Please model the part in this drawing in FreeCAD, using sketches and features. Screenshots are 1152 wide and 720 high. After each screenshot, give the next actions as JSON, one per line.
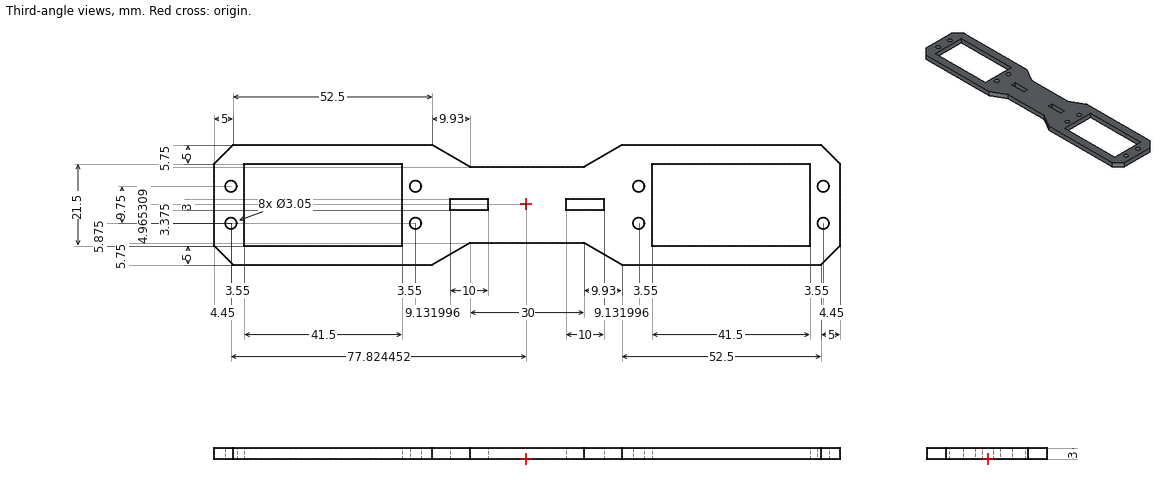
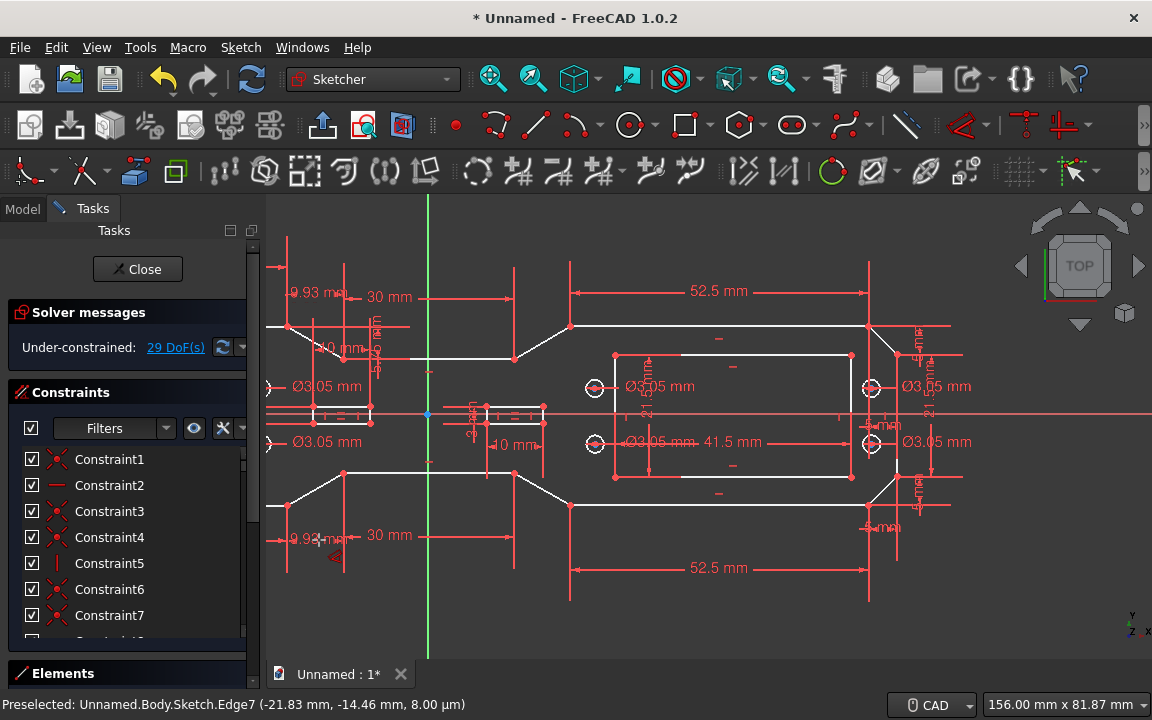
{"action": "left_click", "coordinate": [304, 496]}
{"action": "left_click", "coordinate": [378, 489]}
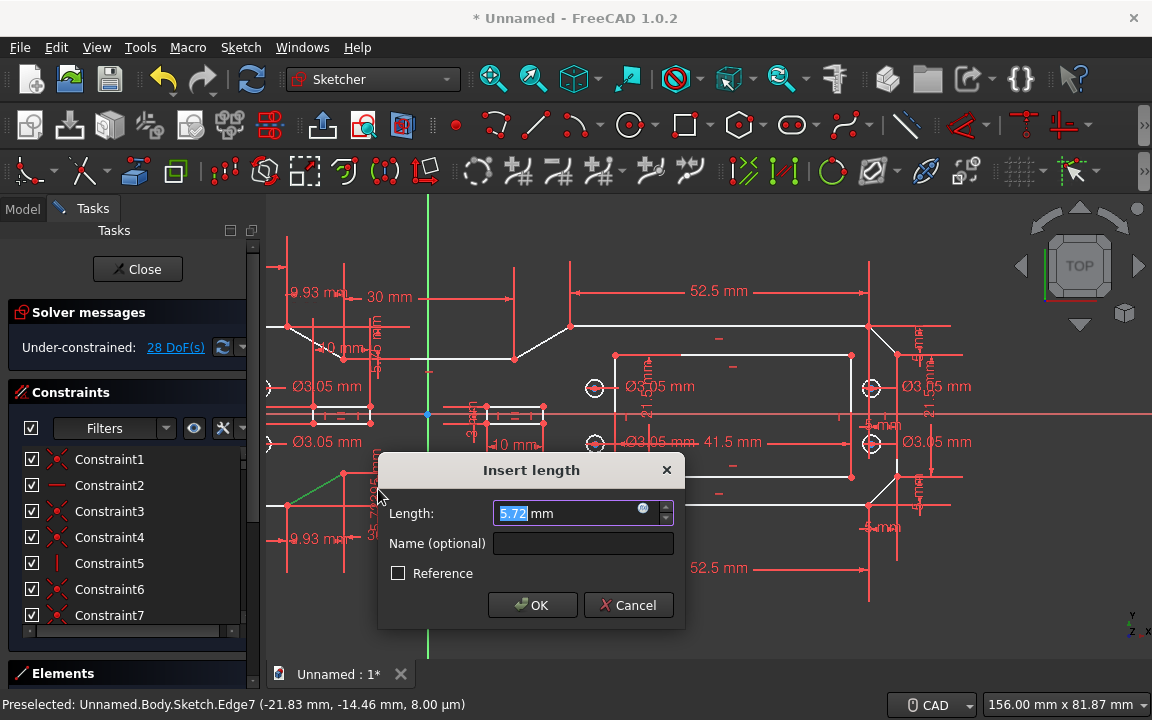
{"action": "type", "text": "5.75"}
{"action": "key", "text": "Return"}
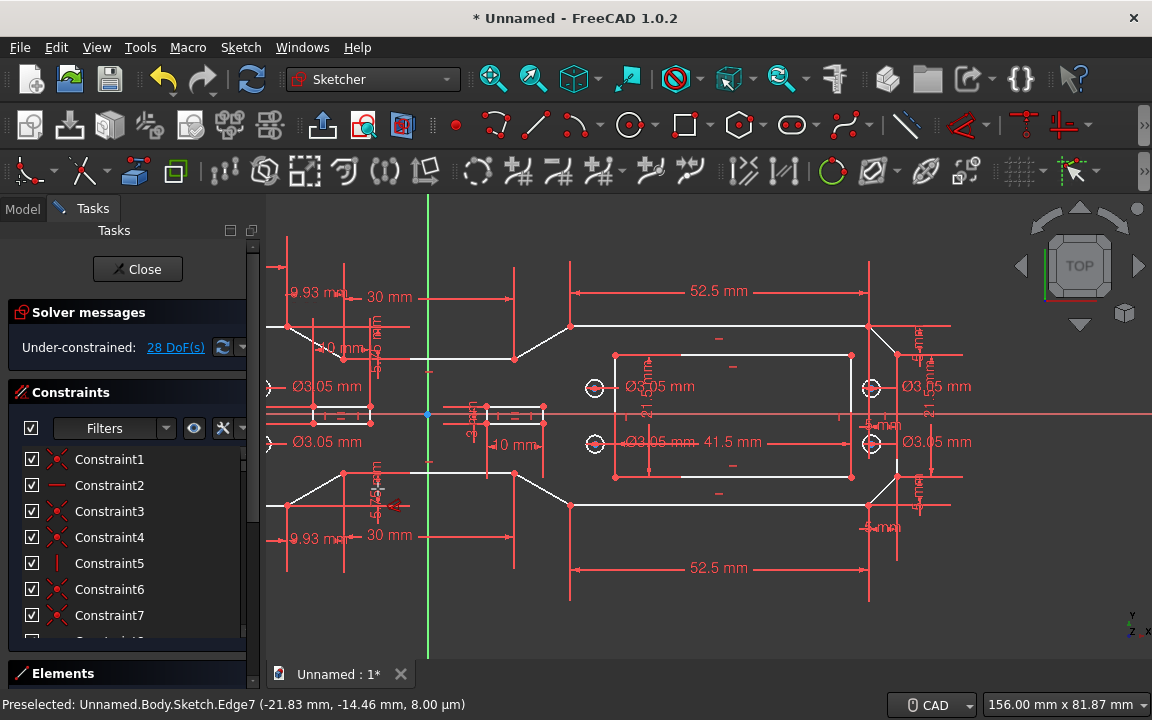
{"action": "left_click", "coordinate": [531, 483]}
{"action": "left_click", "coordinate": [542, 539]}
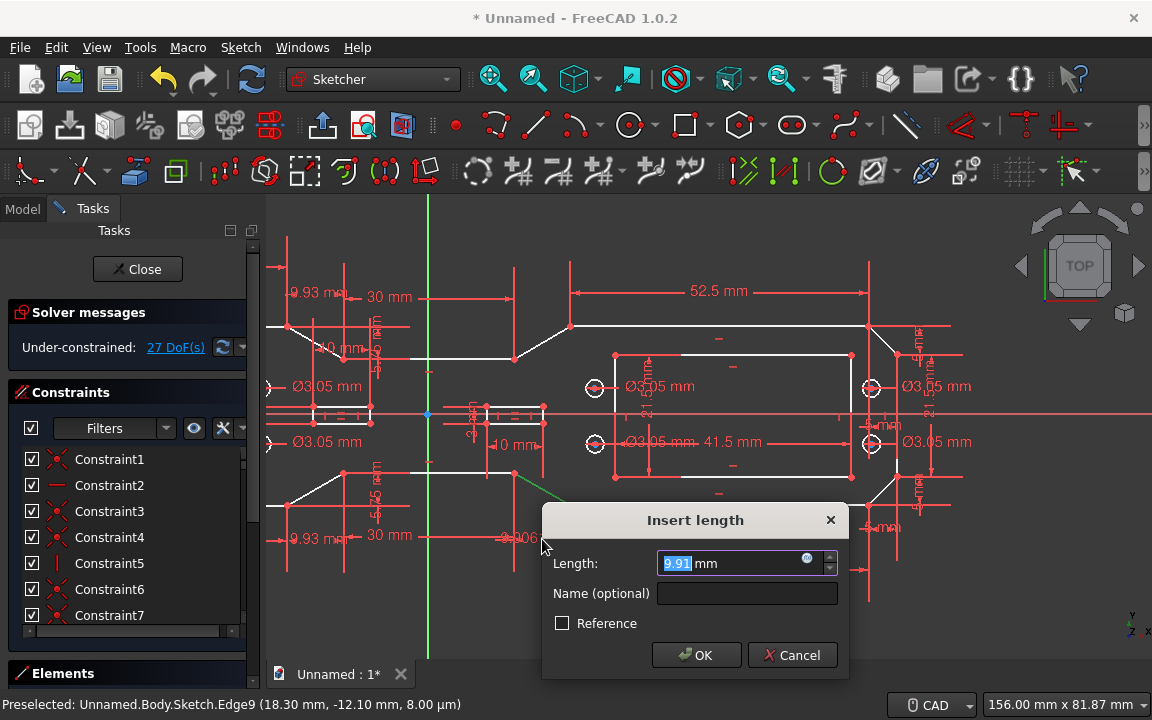
{"action": "type", "text": "9.93"}
{"action": "key", "text": "Return"}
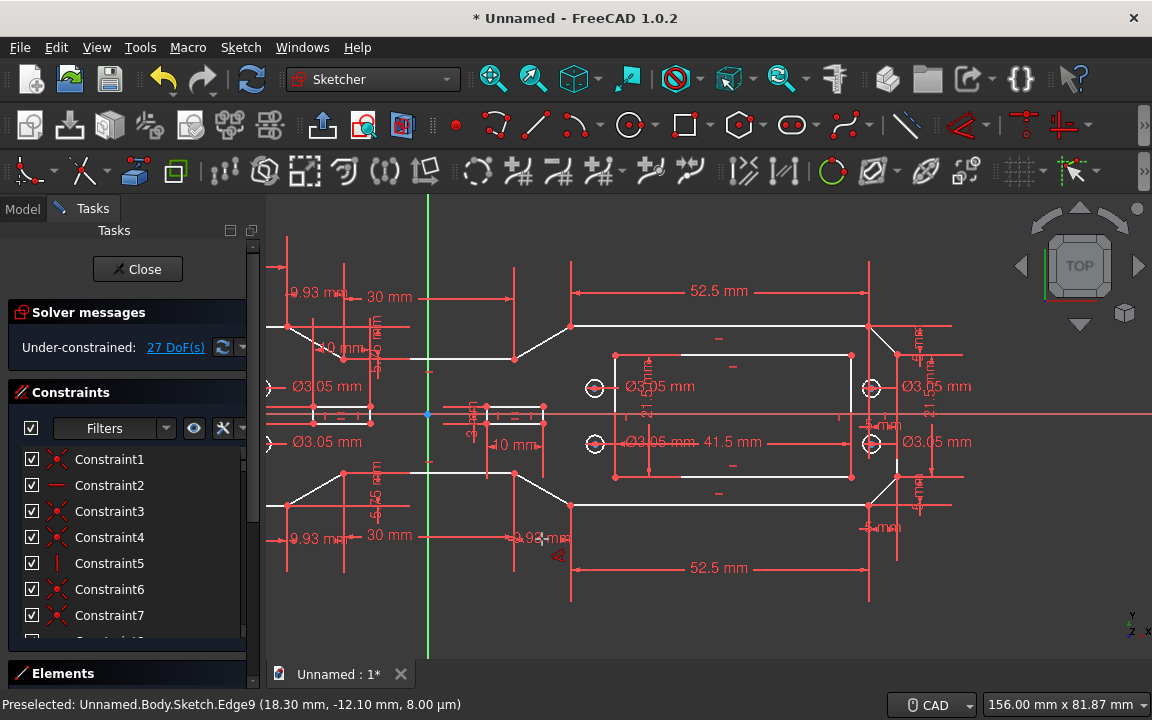
{"action": "left_click", "coordinate": [531, 483]}
{"action": "left_click", "coordinate": [605, 489]}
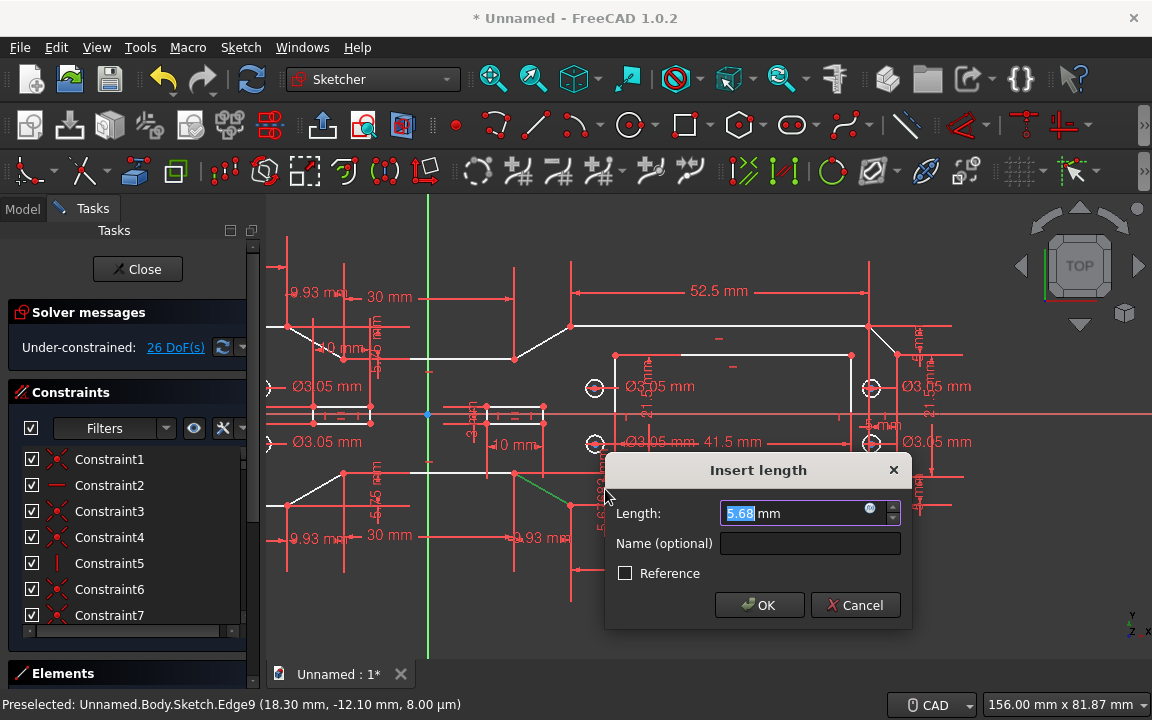
{"action": "type", "text": "5.75"}
{"action": "key", "text": "Return"}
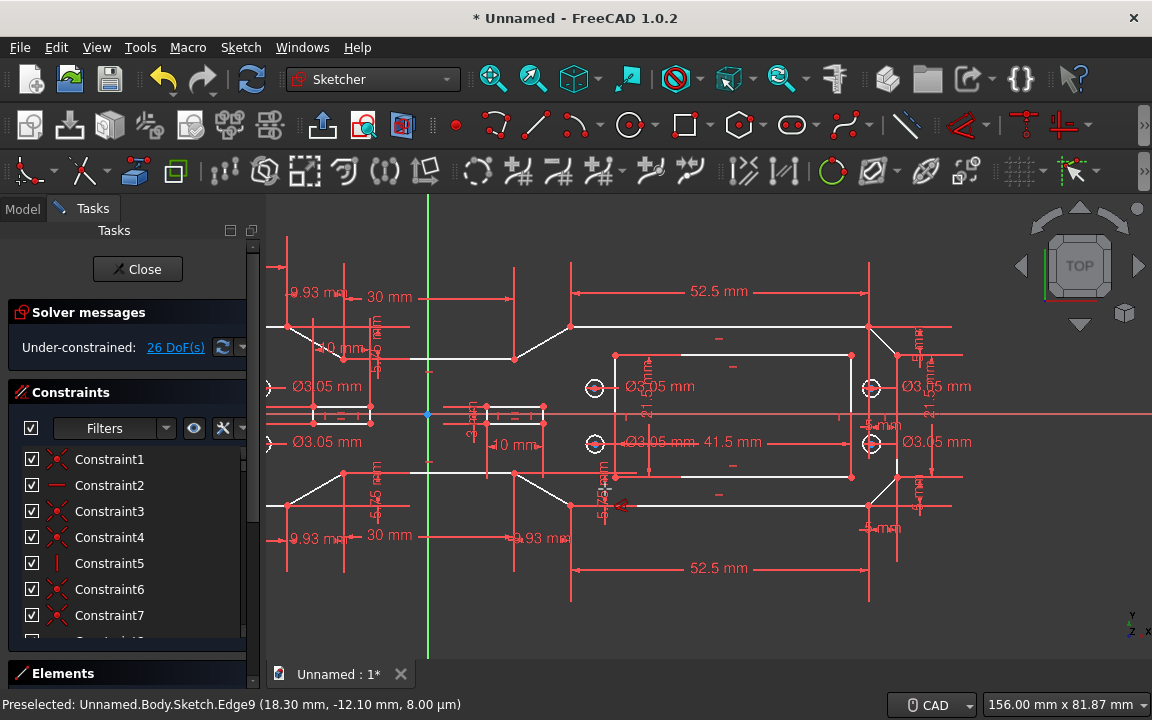
{"action": "scroll", "coordinate": [898, 441], "scroll_direction": "down", "scroll_amount": 3}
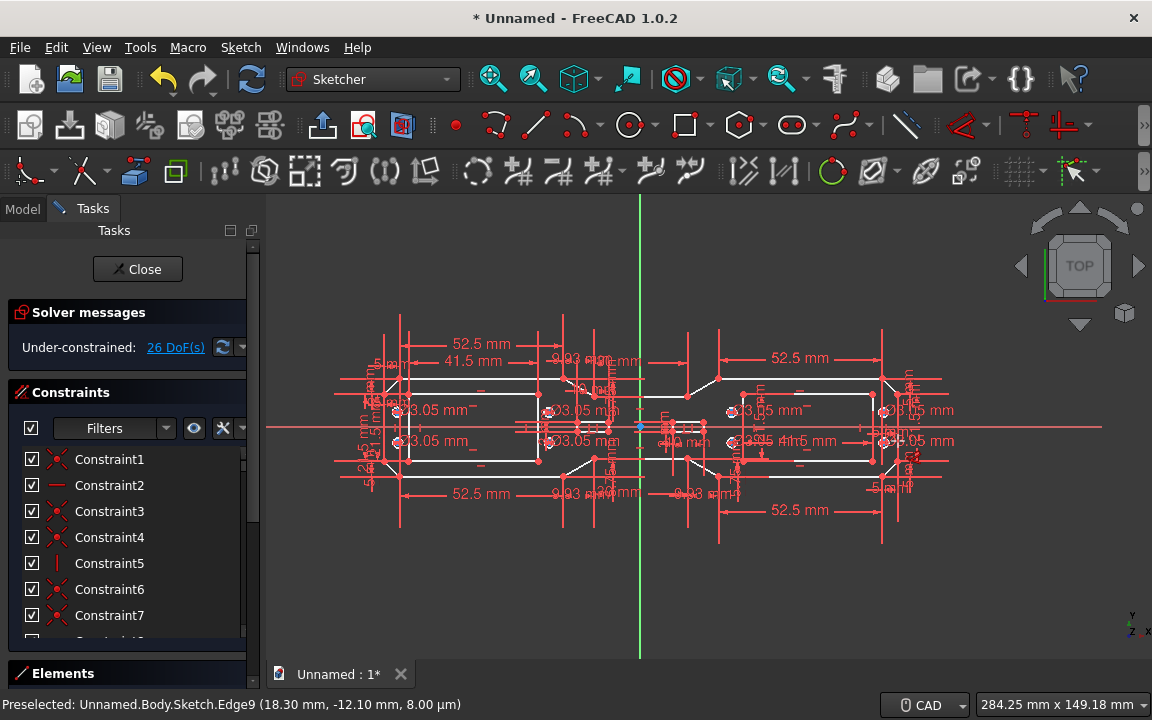
{"action": "scroll", "coordinate": [409, 461], "scroll_direction": "up", "scroll_amount": 7}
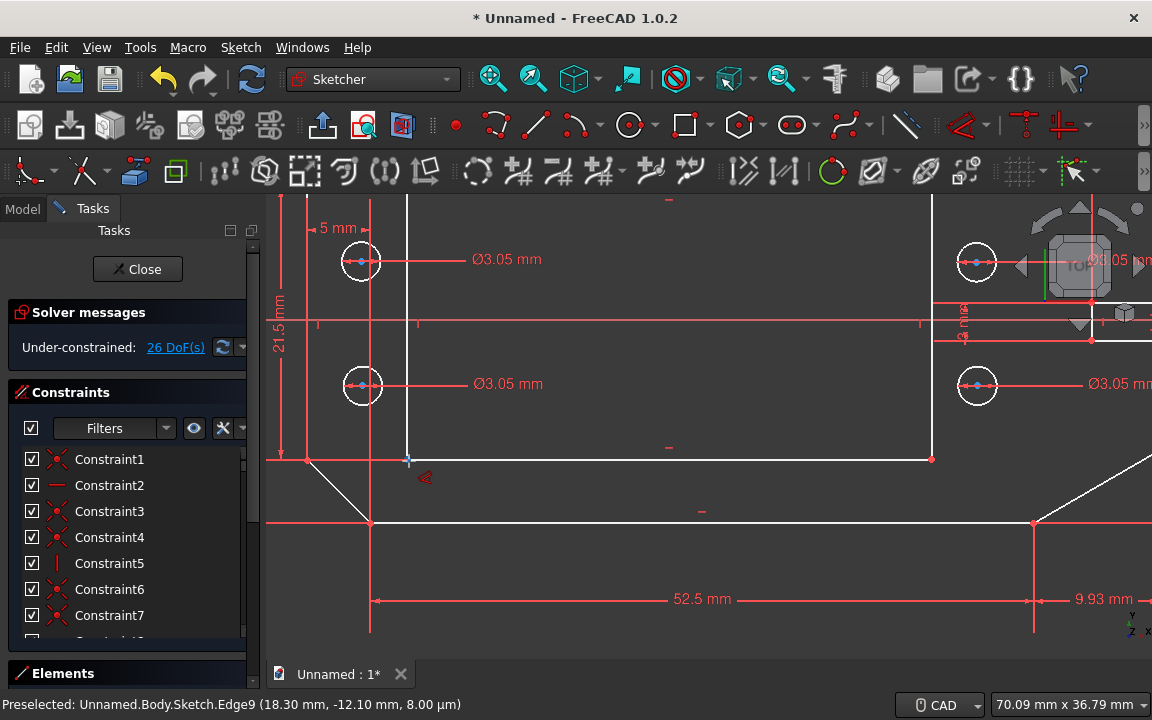
{"action": "left_click", "coordinate": [407, 460]}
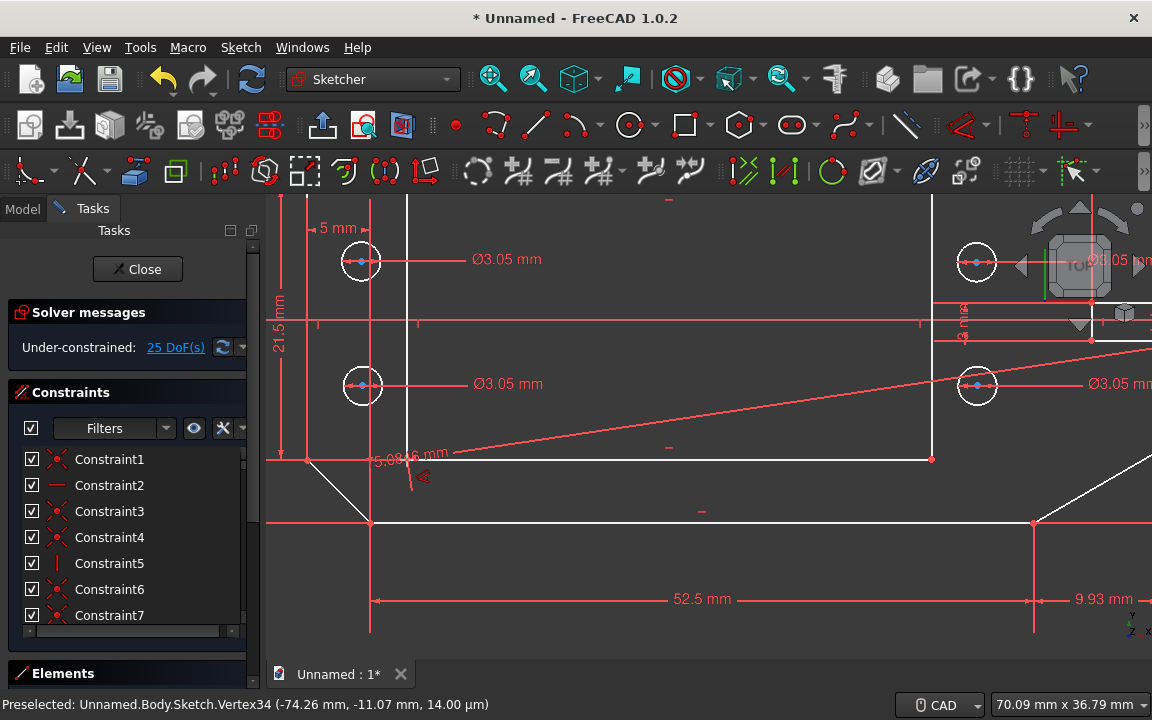
{"action": "left_click", "coordinate": [363, 386]}
{"action": "left_click", "coordinate": [385, 494]}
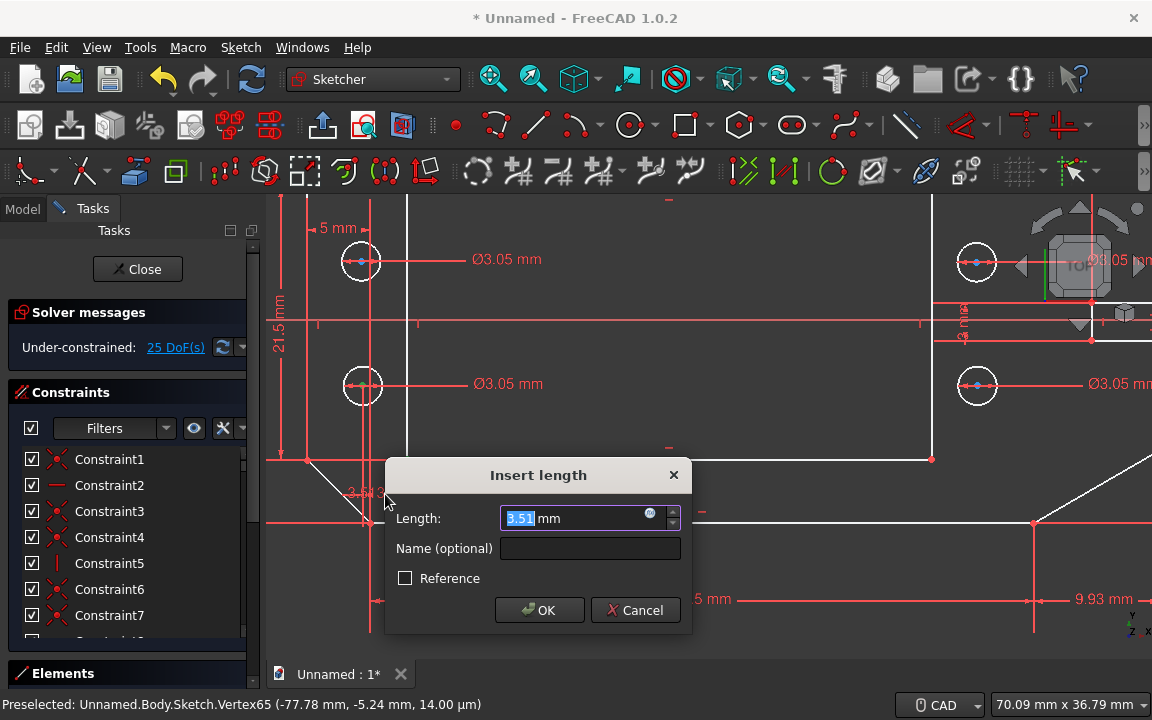
{"action": "type", "text": "3.55"}
{"action": "key", "text": "Return"}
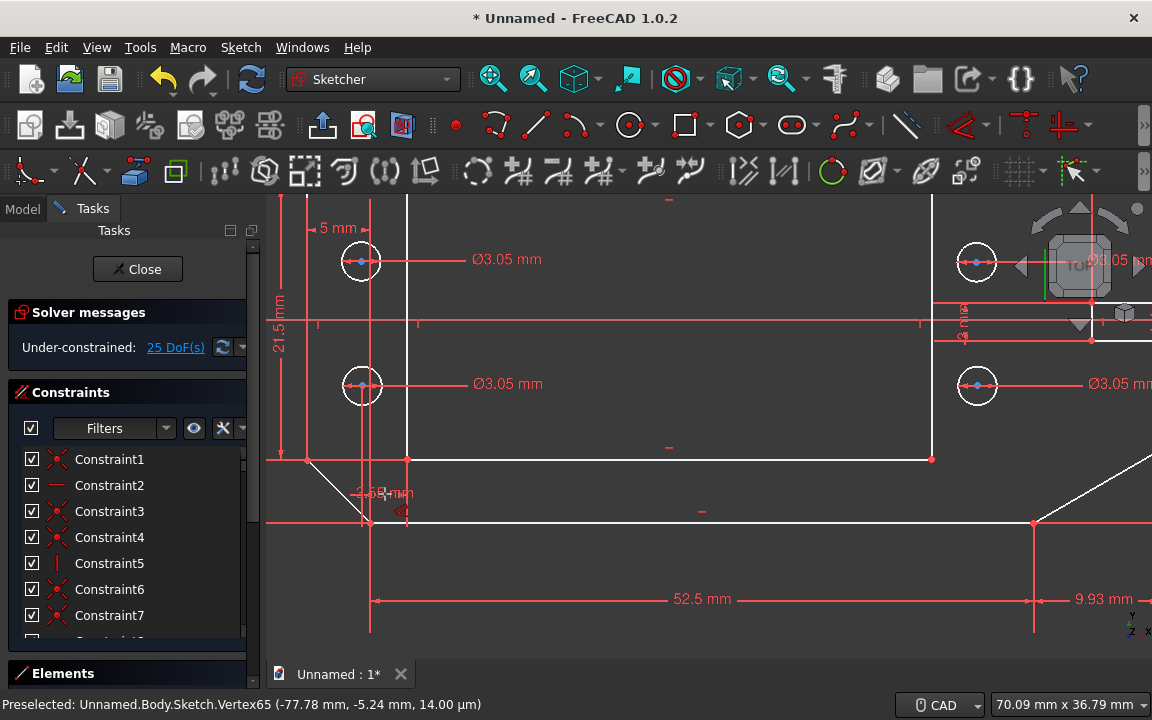
{"action": "left_click", "coordinate": [307, 460]}